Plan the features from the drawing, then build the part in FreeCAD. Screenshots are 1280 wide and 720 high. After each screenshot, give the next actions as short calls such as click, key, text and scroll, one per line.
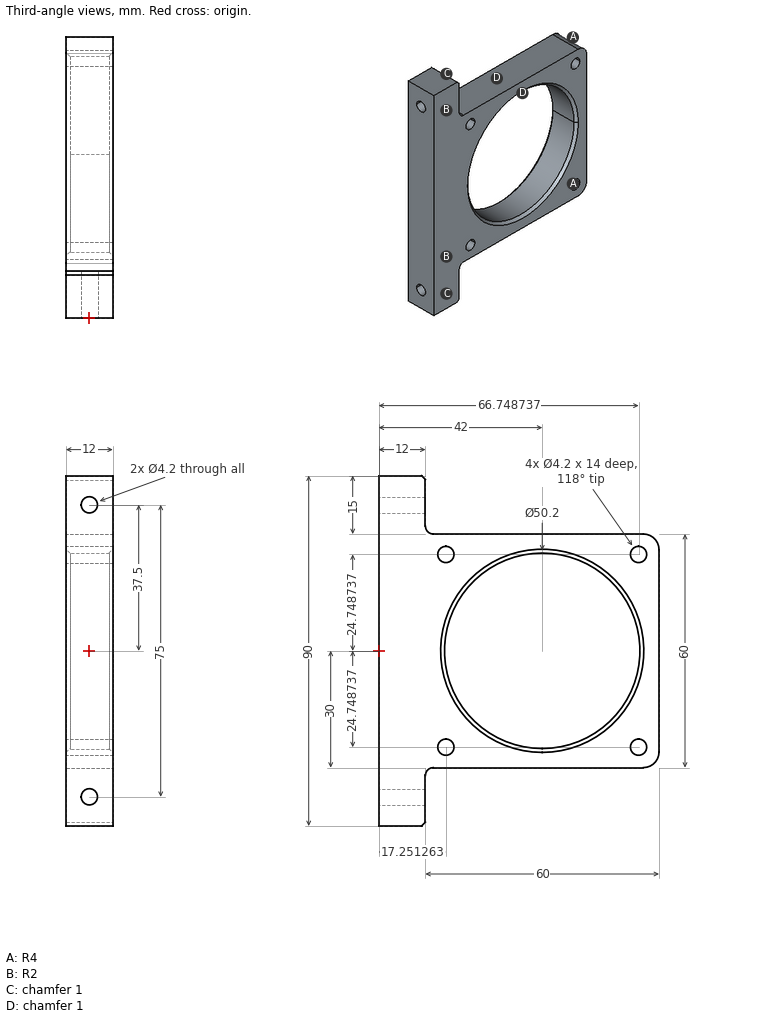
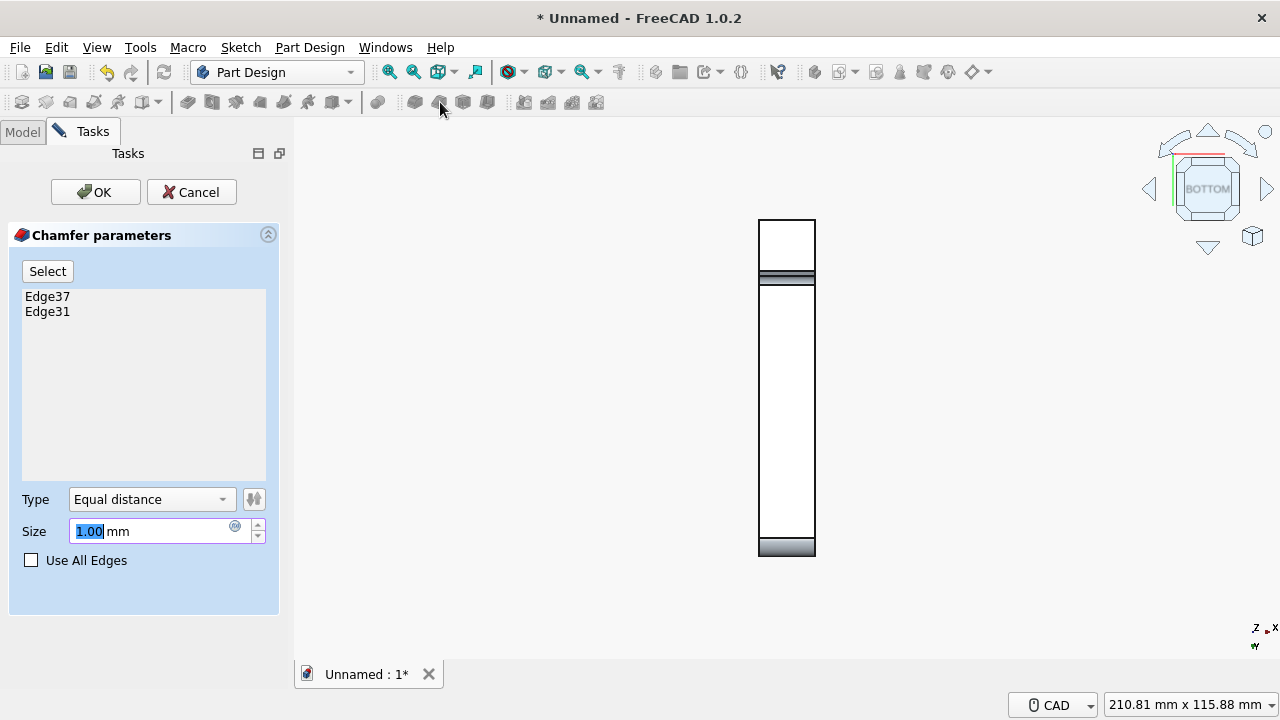
text(1)
key(Tab)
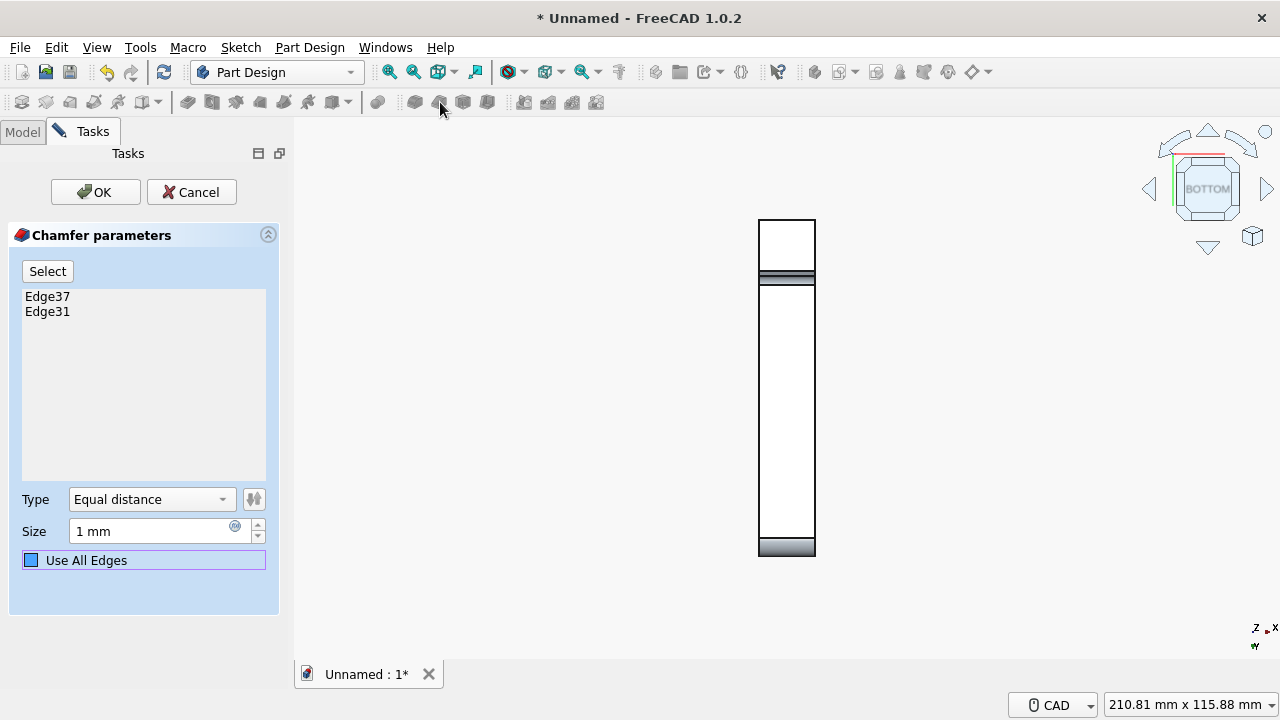
click(96, 192)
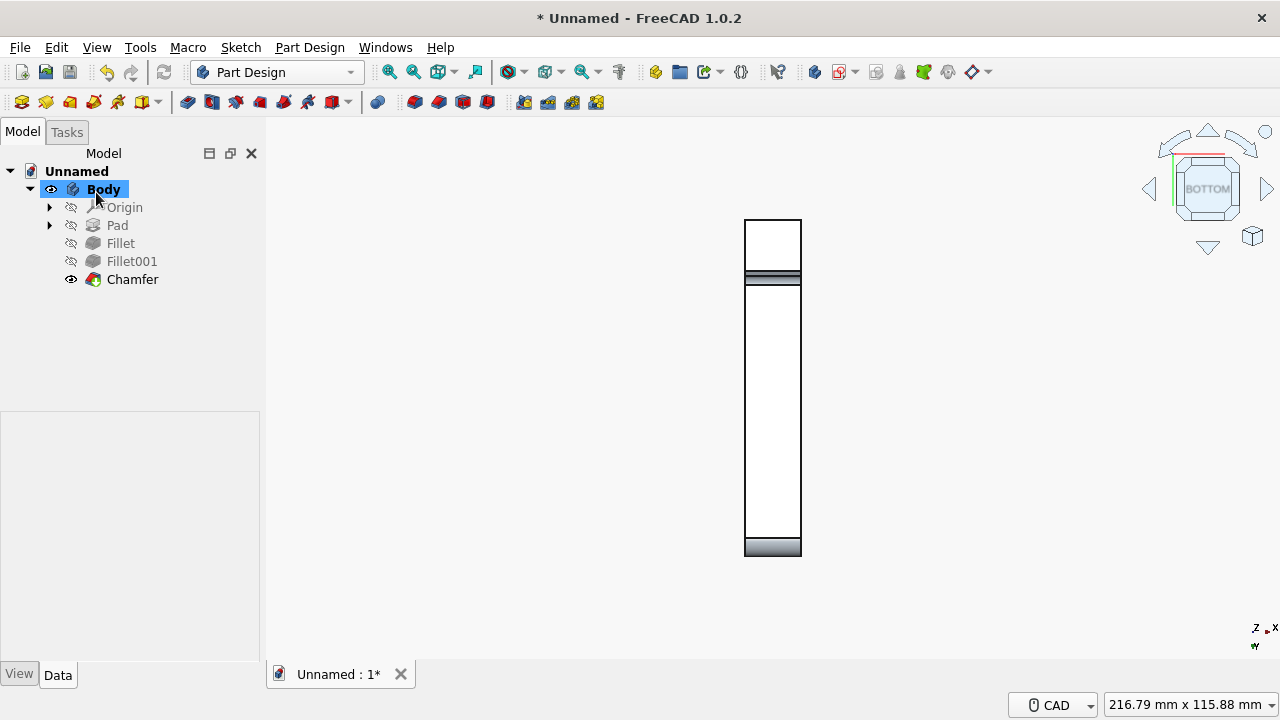
key(4)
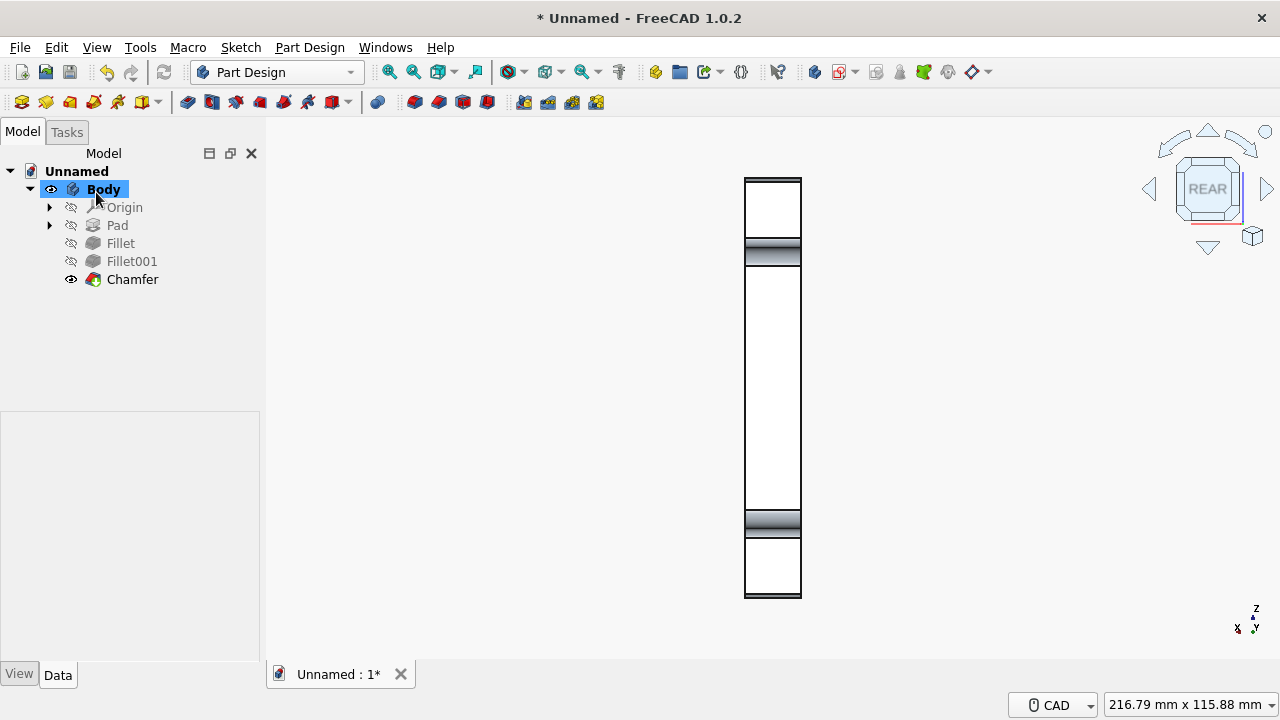
click(773, 565)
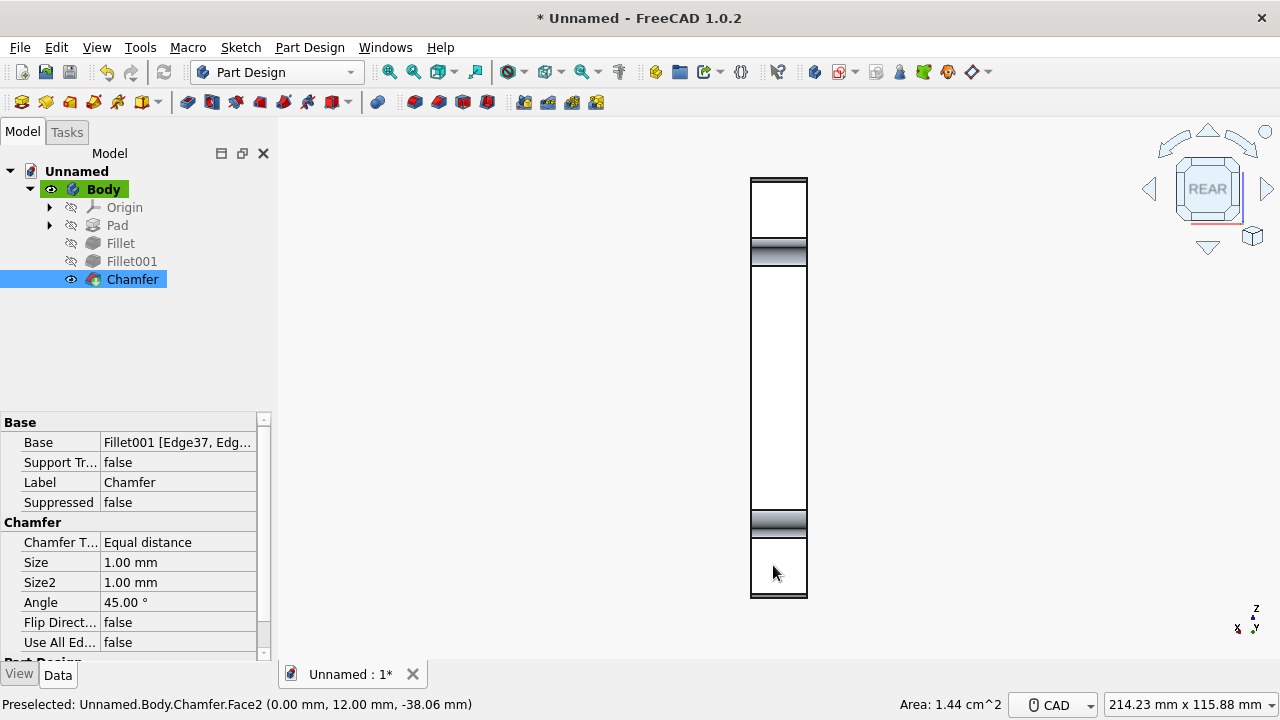
click(840, 72)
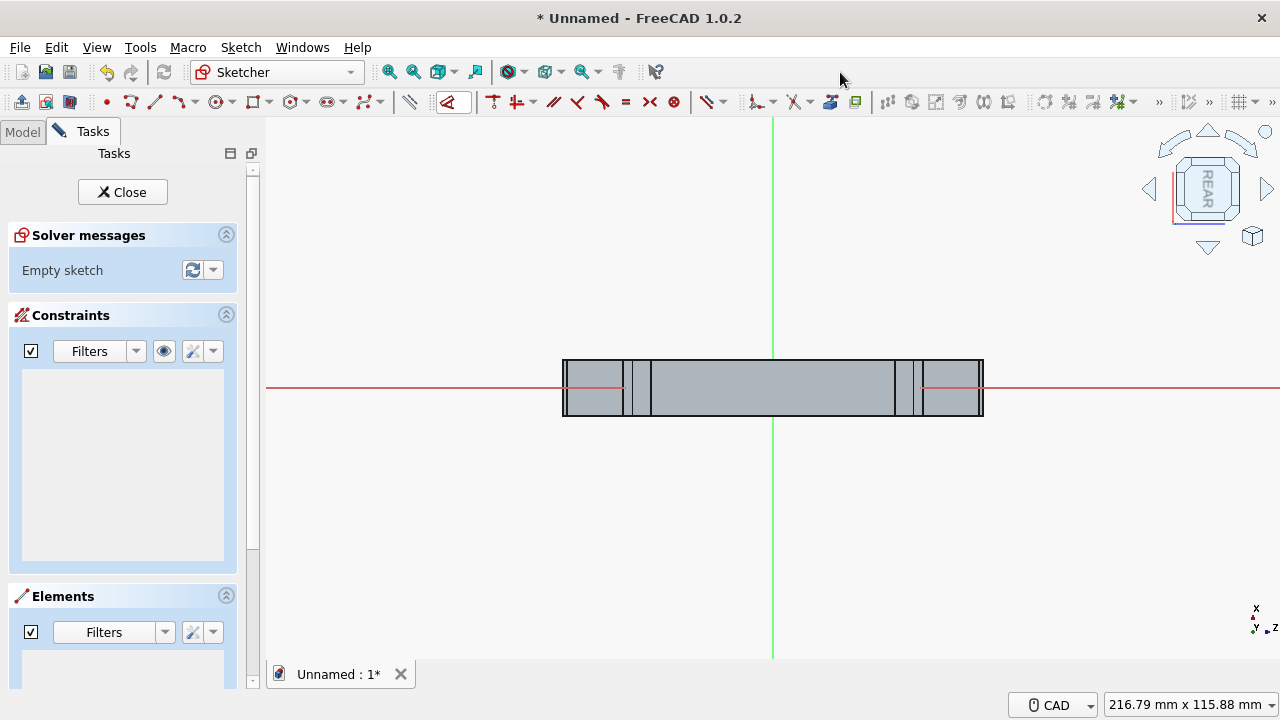
click(70, 102)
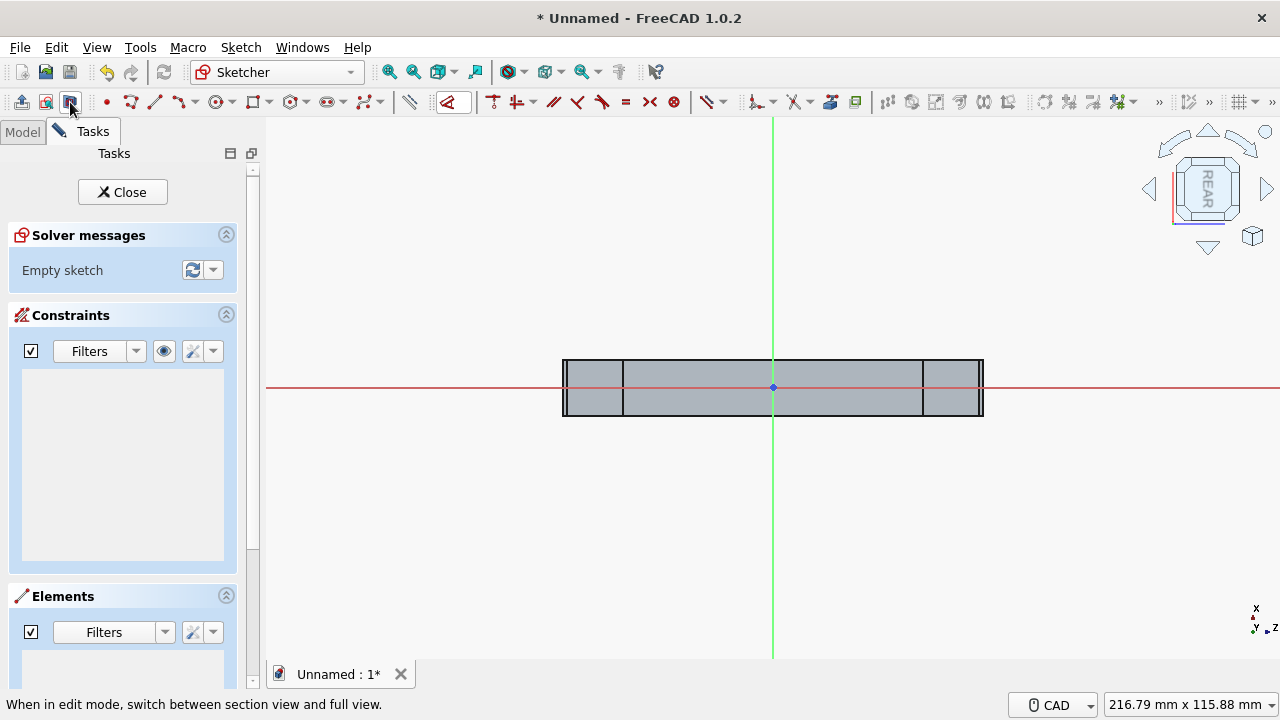
scroll(912, 388, up, 2)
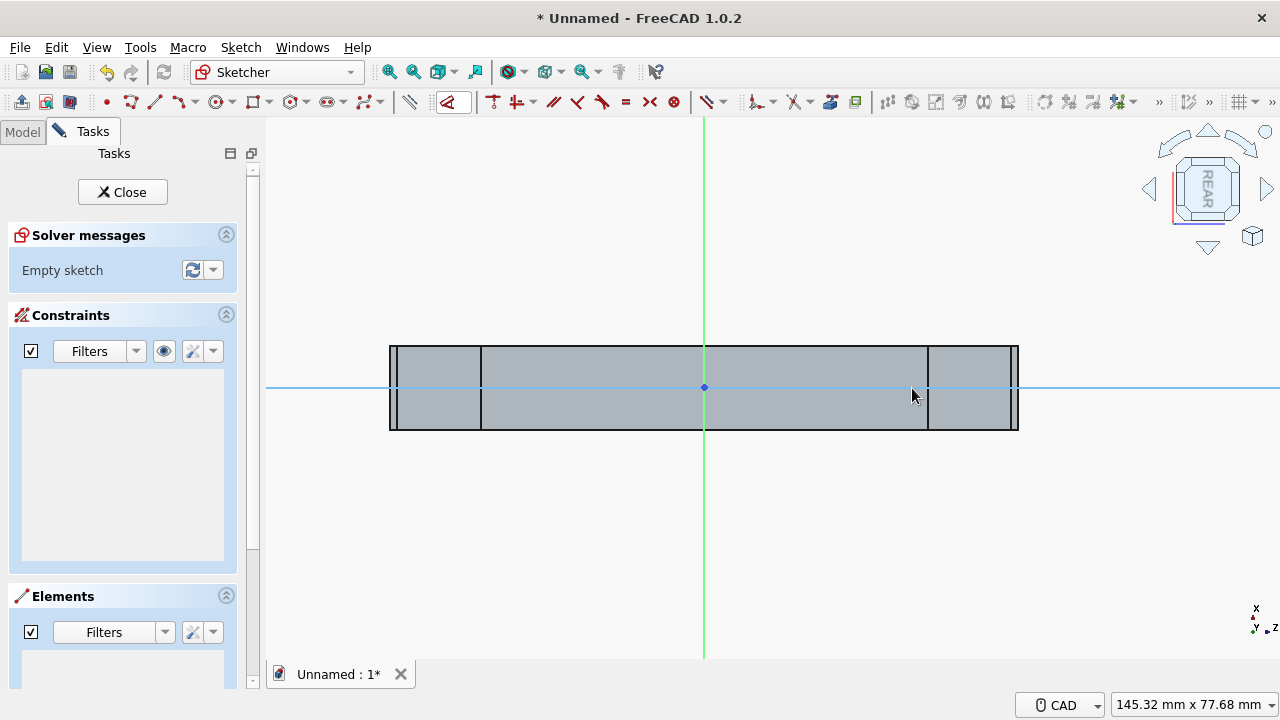
click(216, 102)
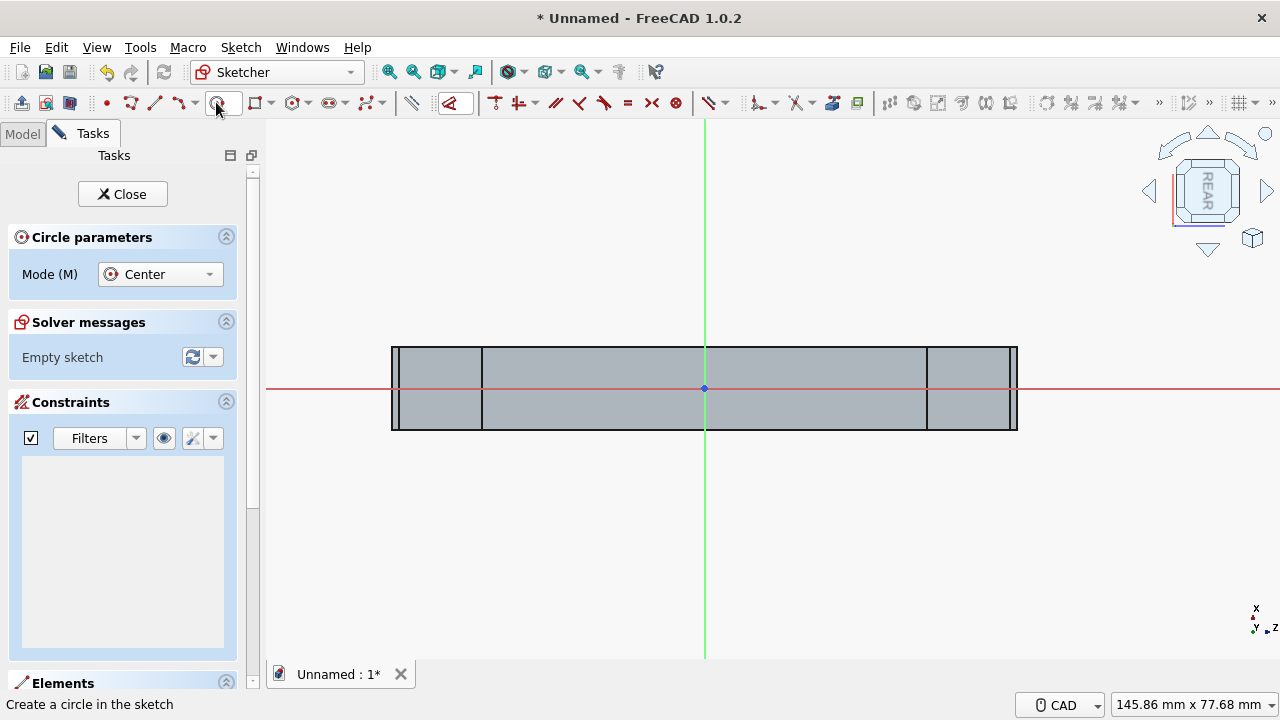
scroll(965, 389, up, 3)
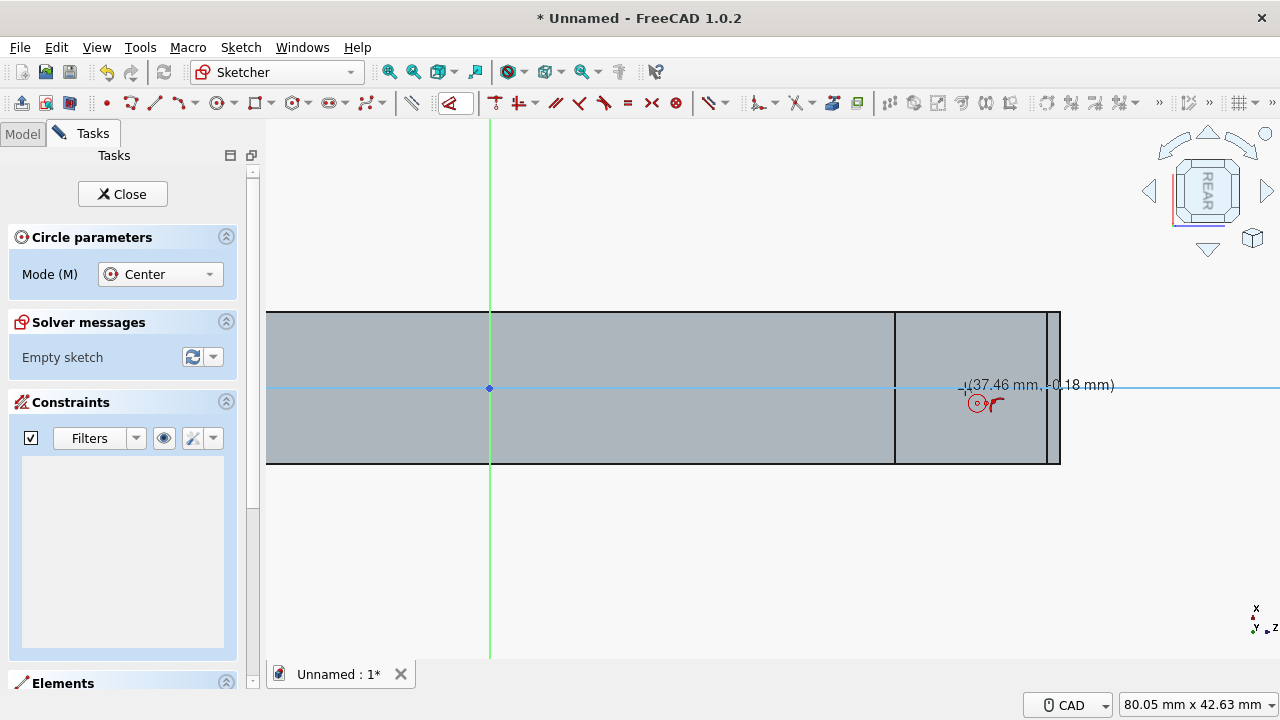
click(965, 388)
move(984, 369)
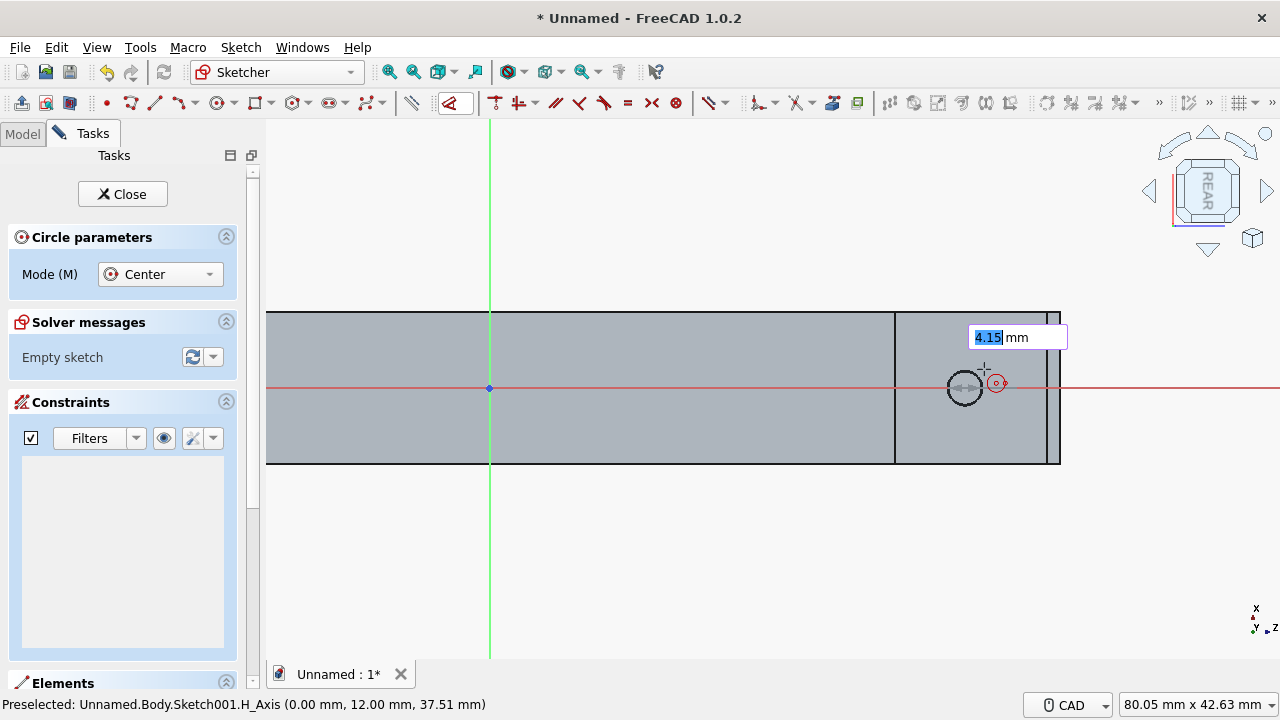
text(4.2)
key(Return)